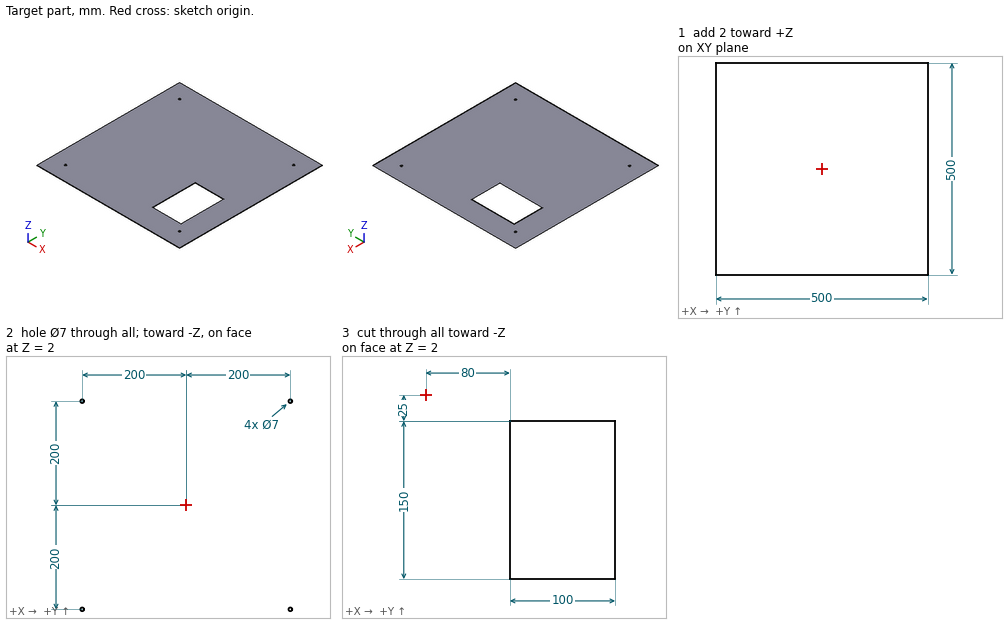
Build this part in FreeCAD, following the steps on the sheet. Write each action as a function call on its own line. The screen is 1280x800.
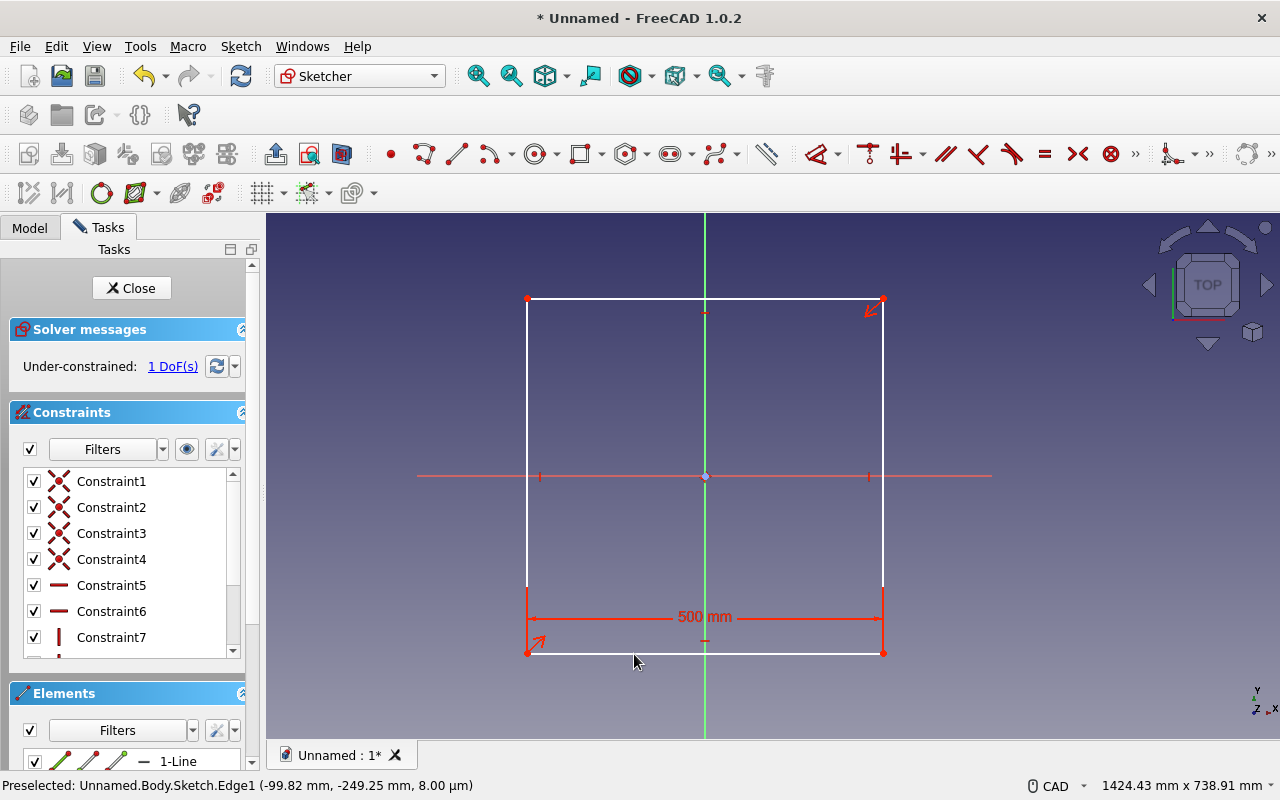
click(883, 547)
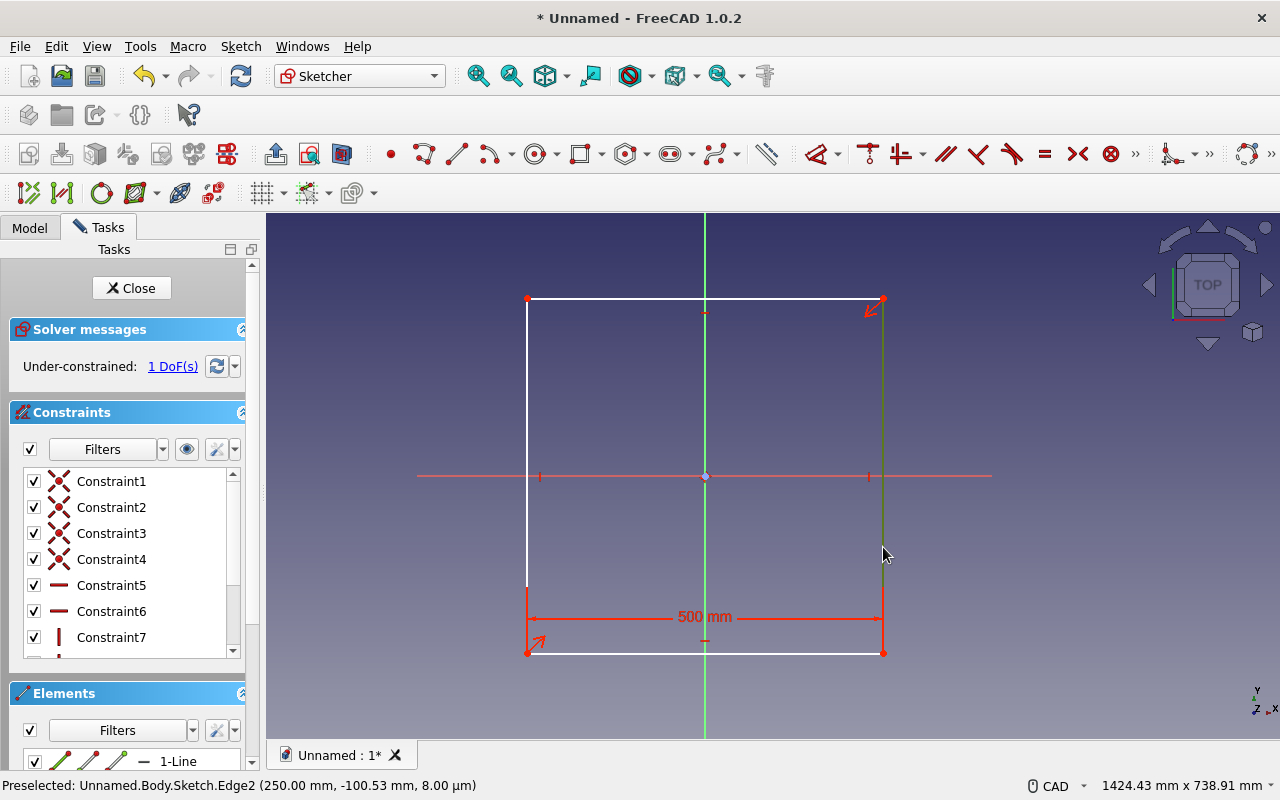
key(i)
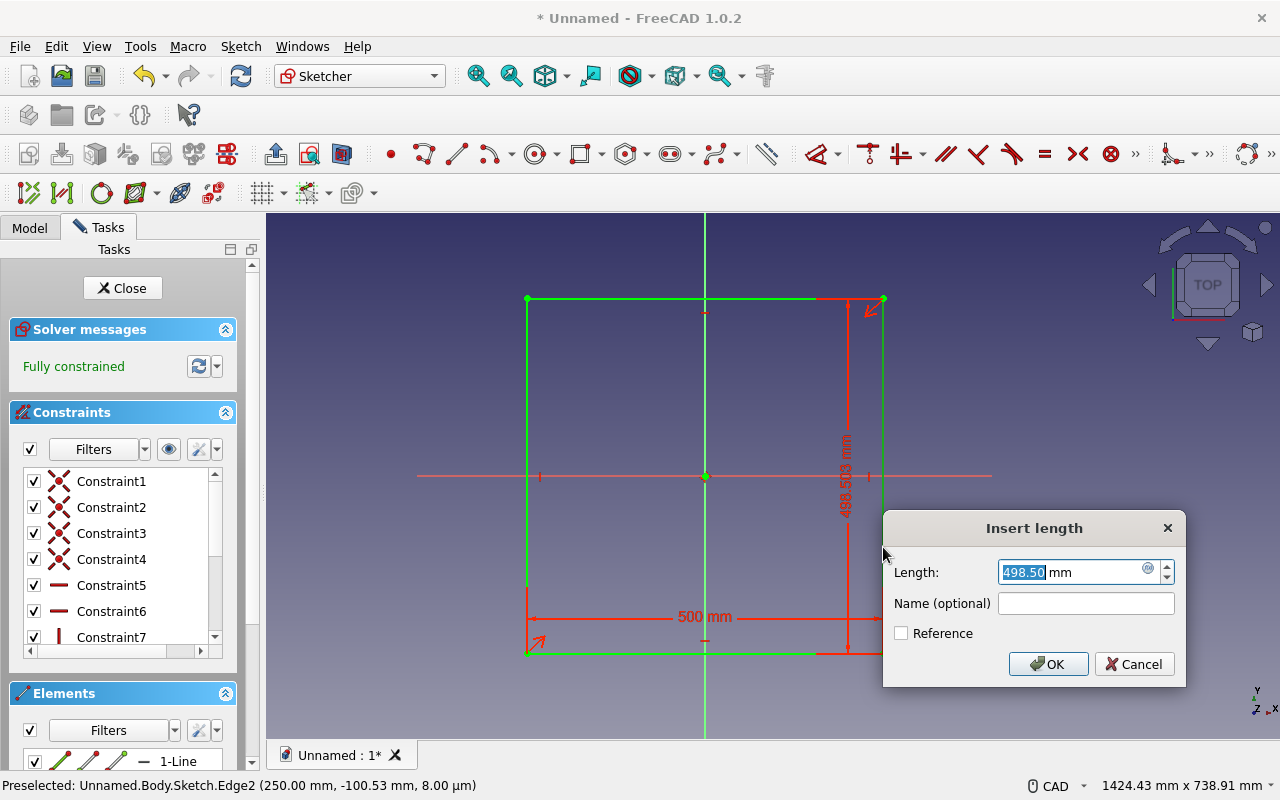
text(500)
key(Return)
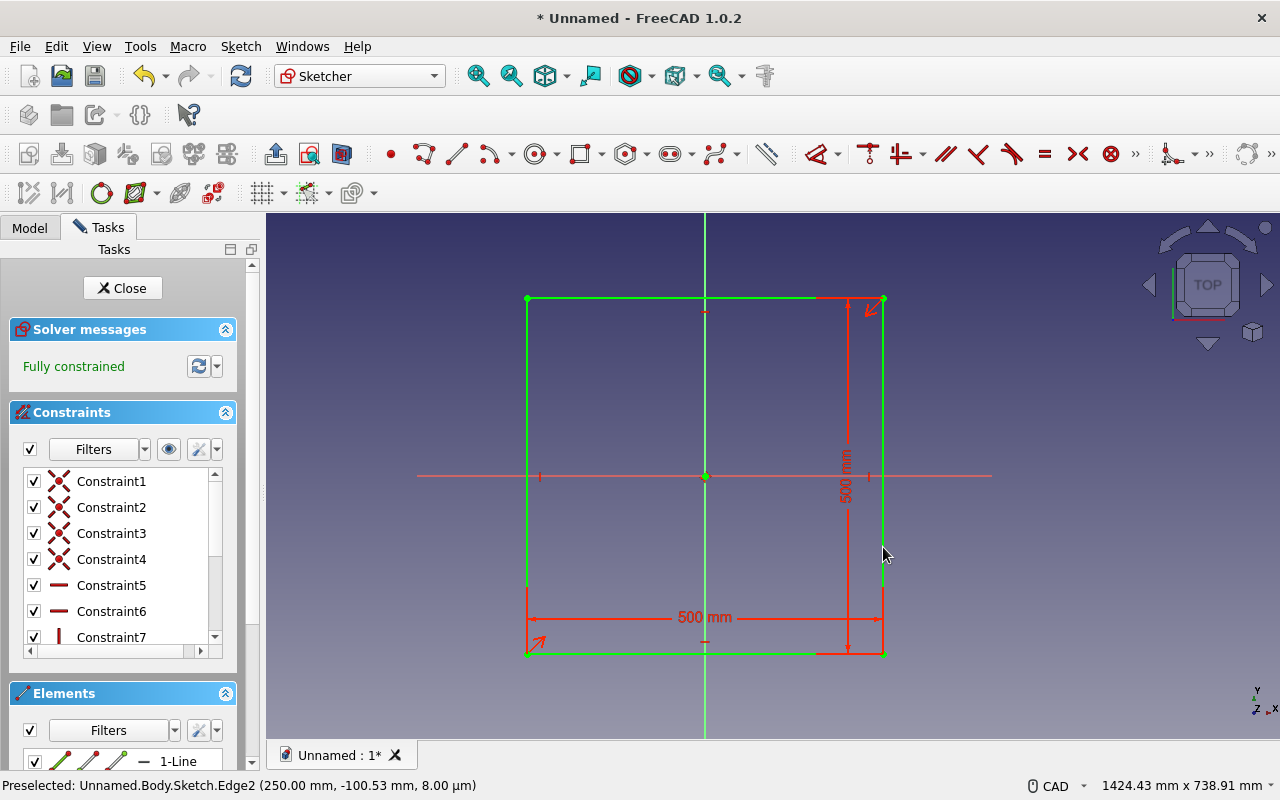
click(123, 288)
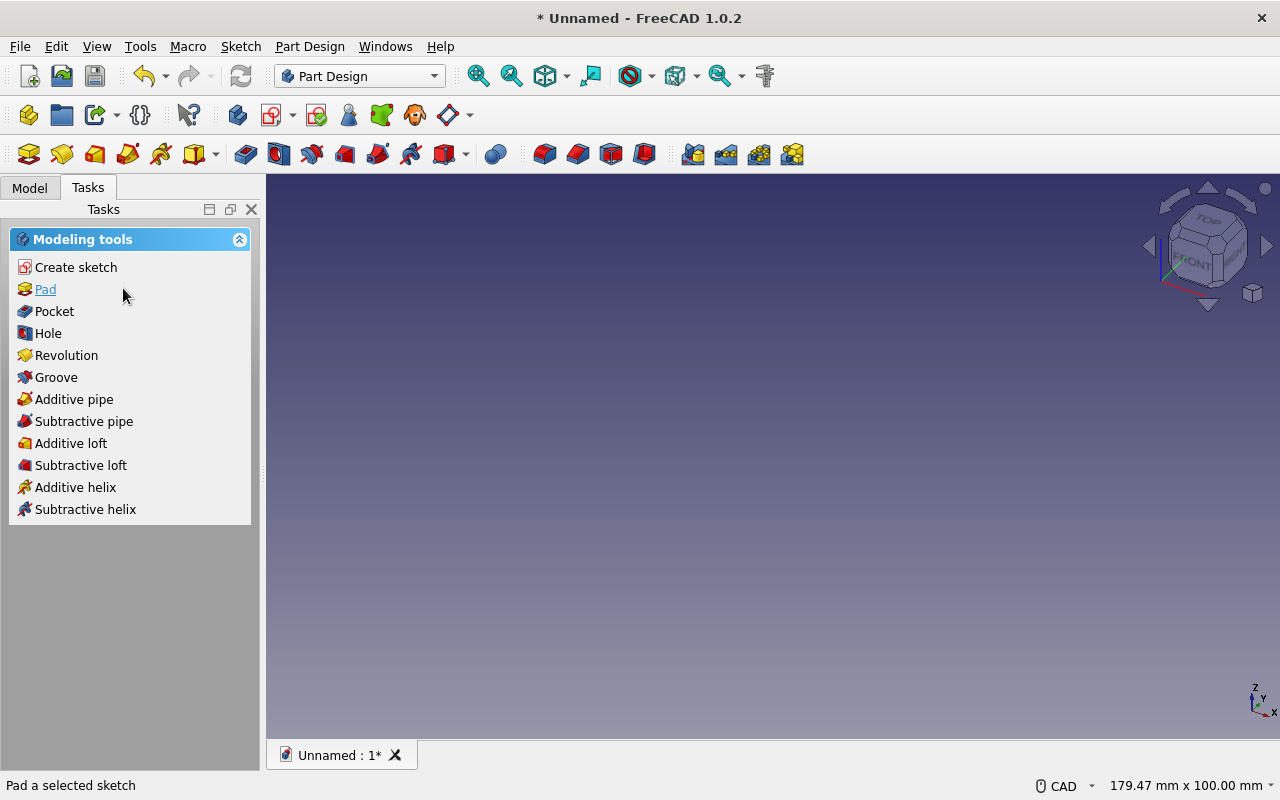
click(29, 154)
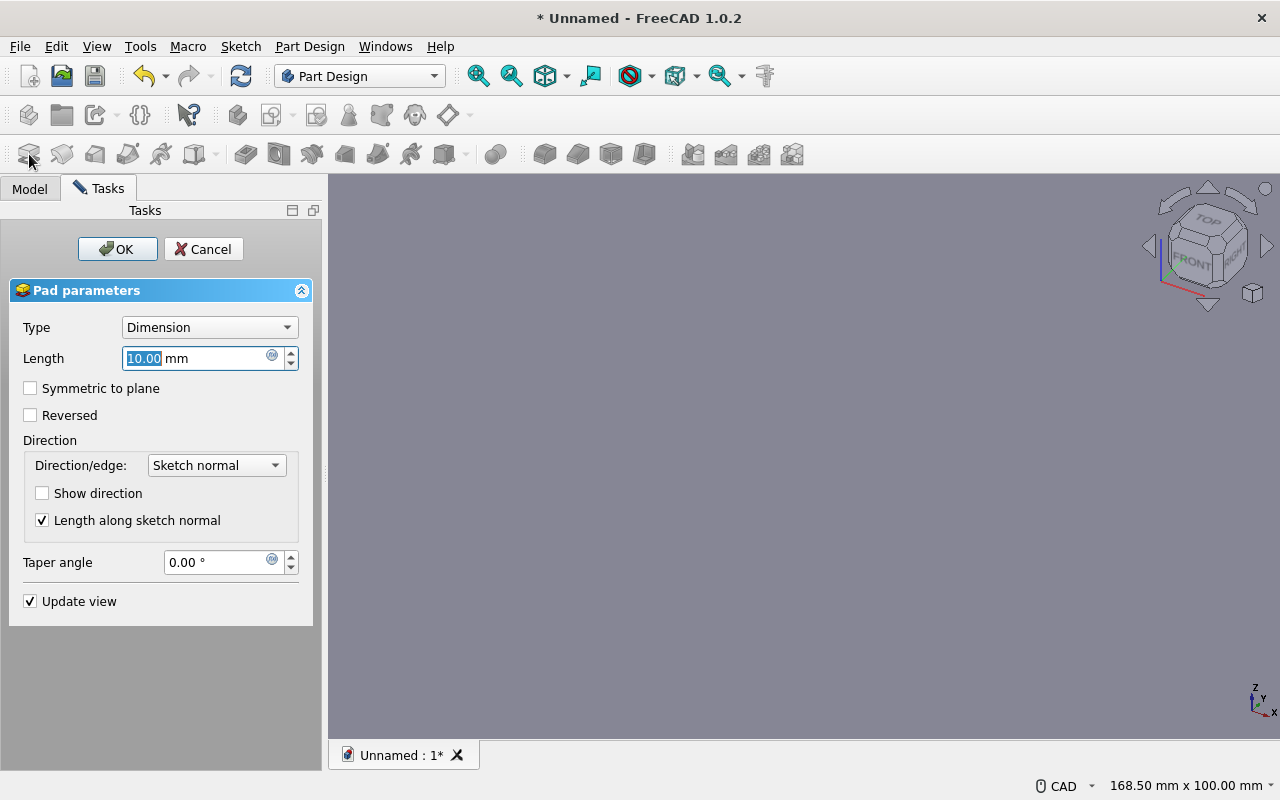
text(2)
key(Tab)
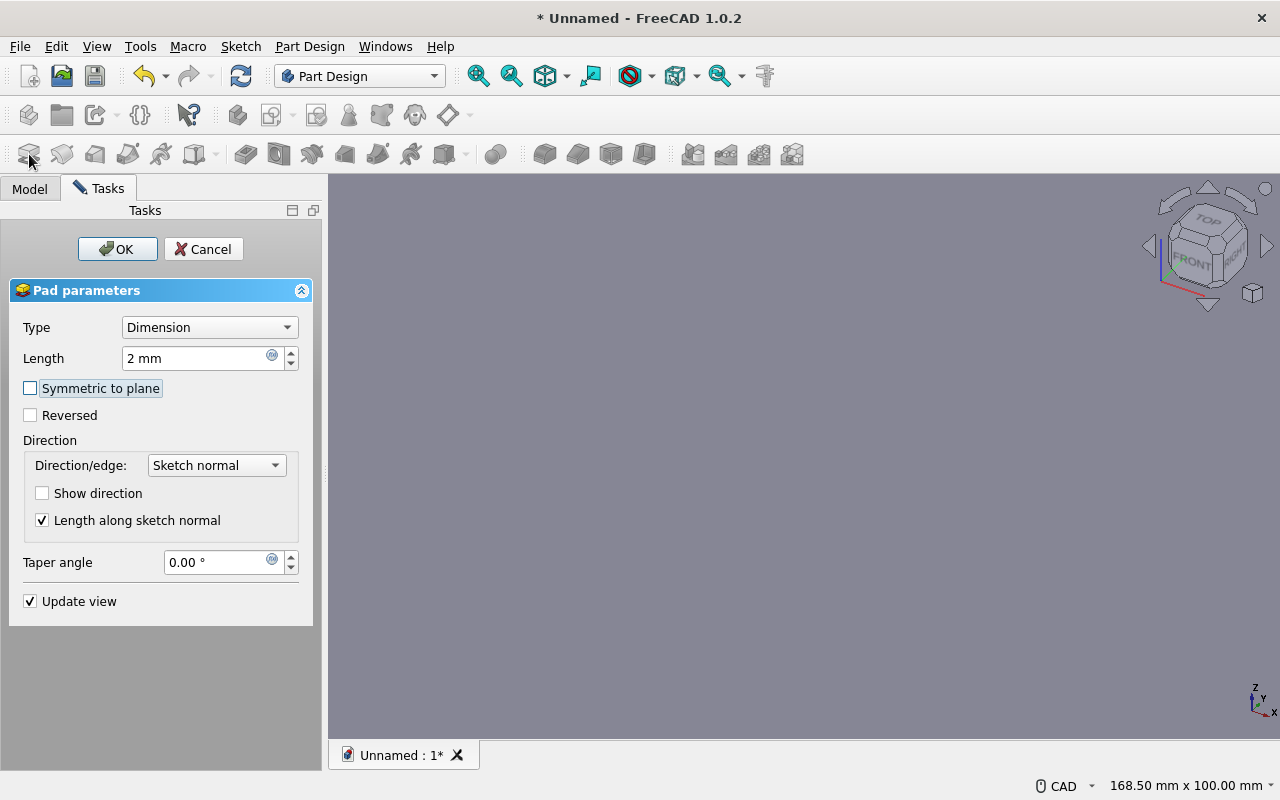
click(118, 249)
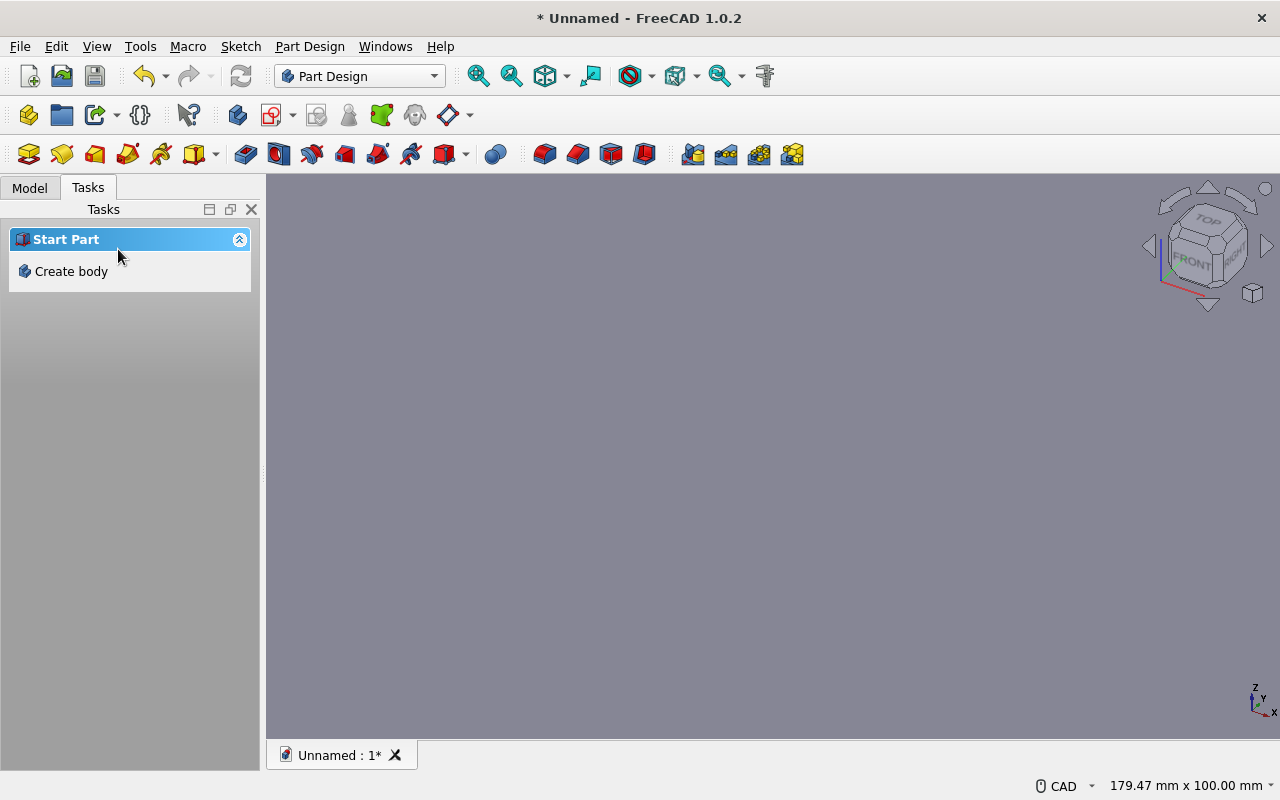
key(v)
key(f)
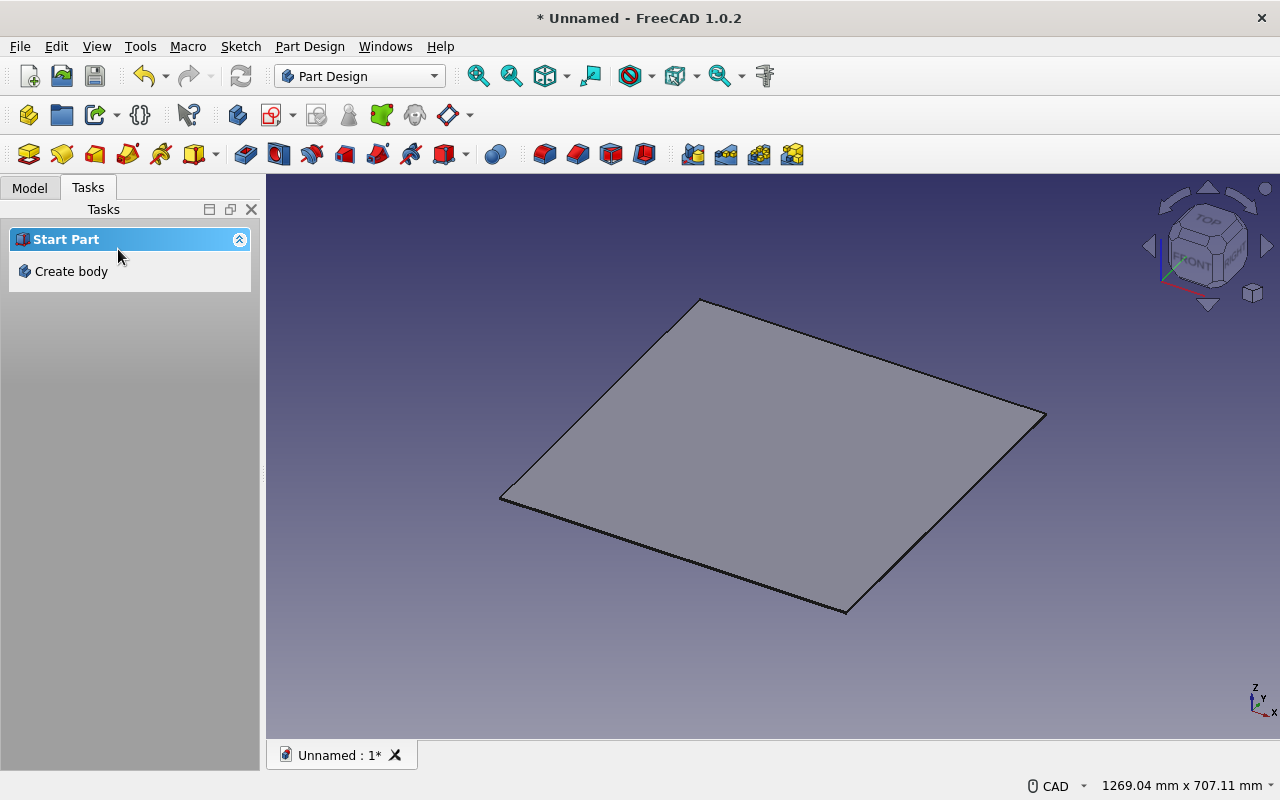
click(773, 455)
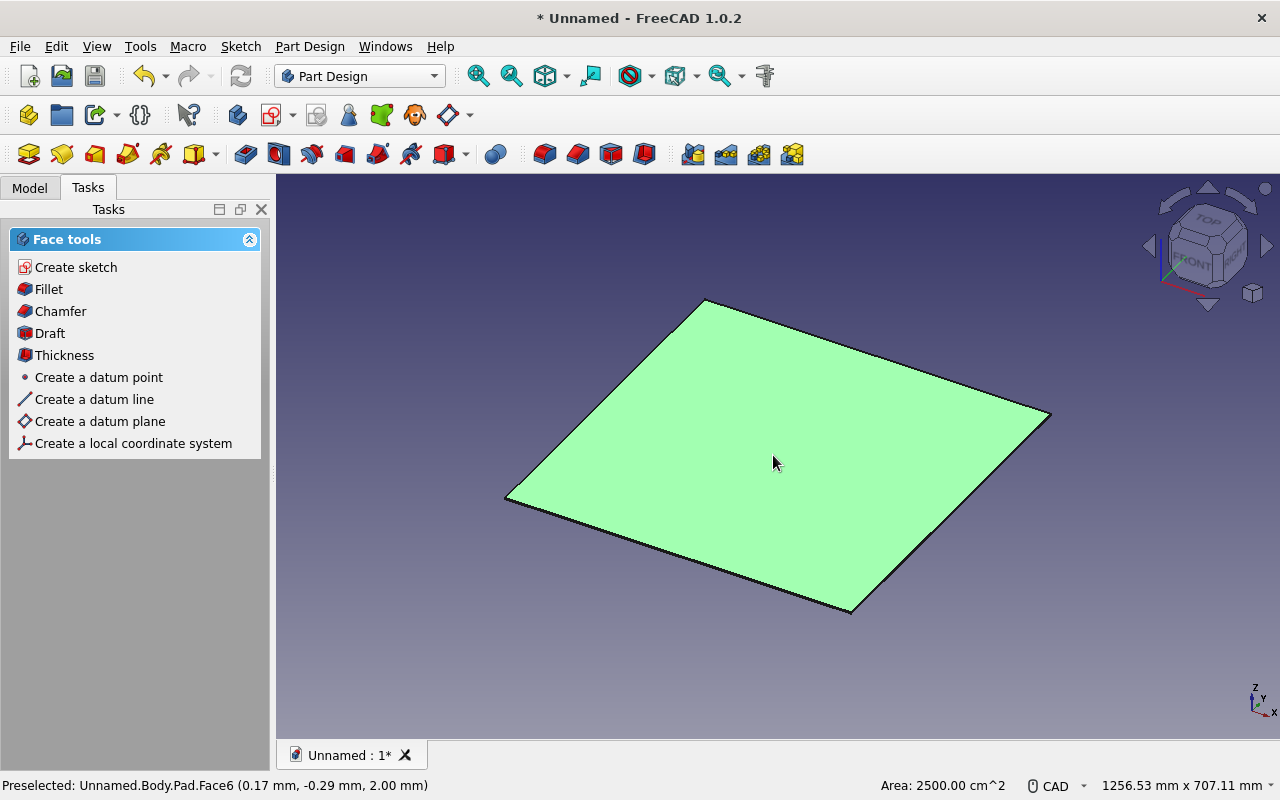
click(270, 116)